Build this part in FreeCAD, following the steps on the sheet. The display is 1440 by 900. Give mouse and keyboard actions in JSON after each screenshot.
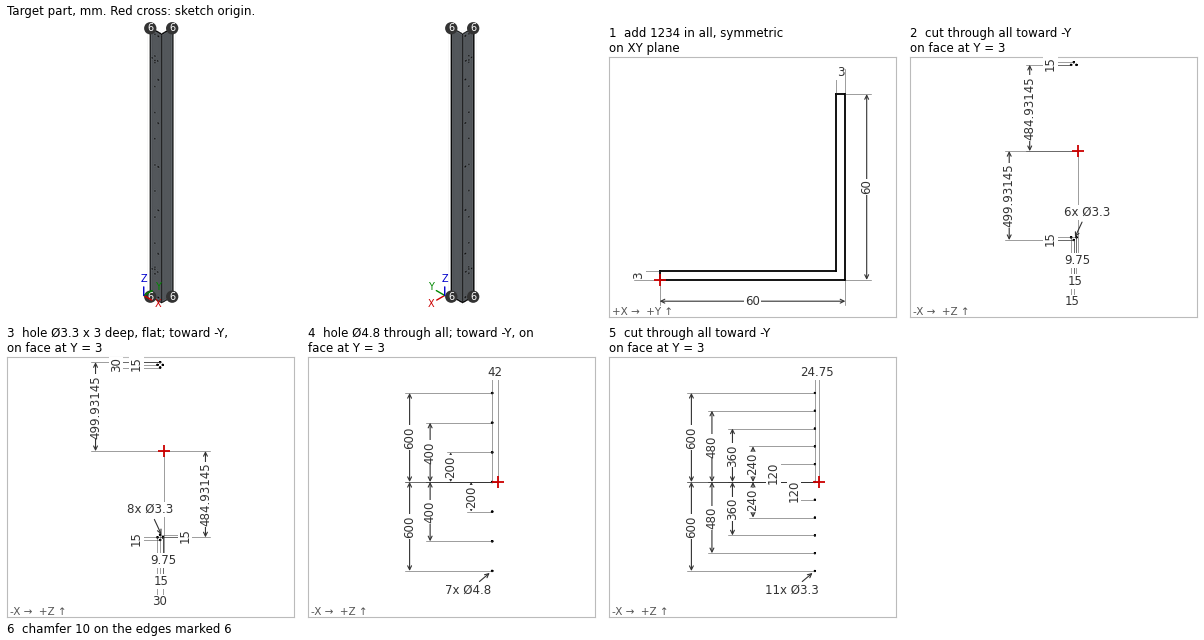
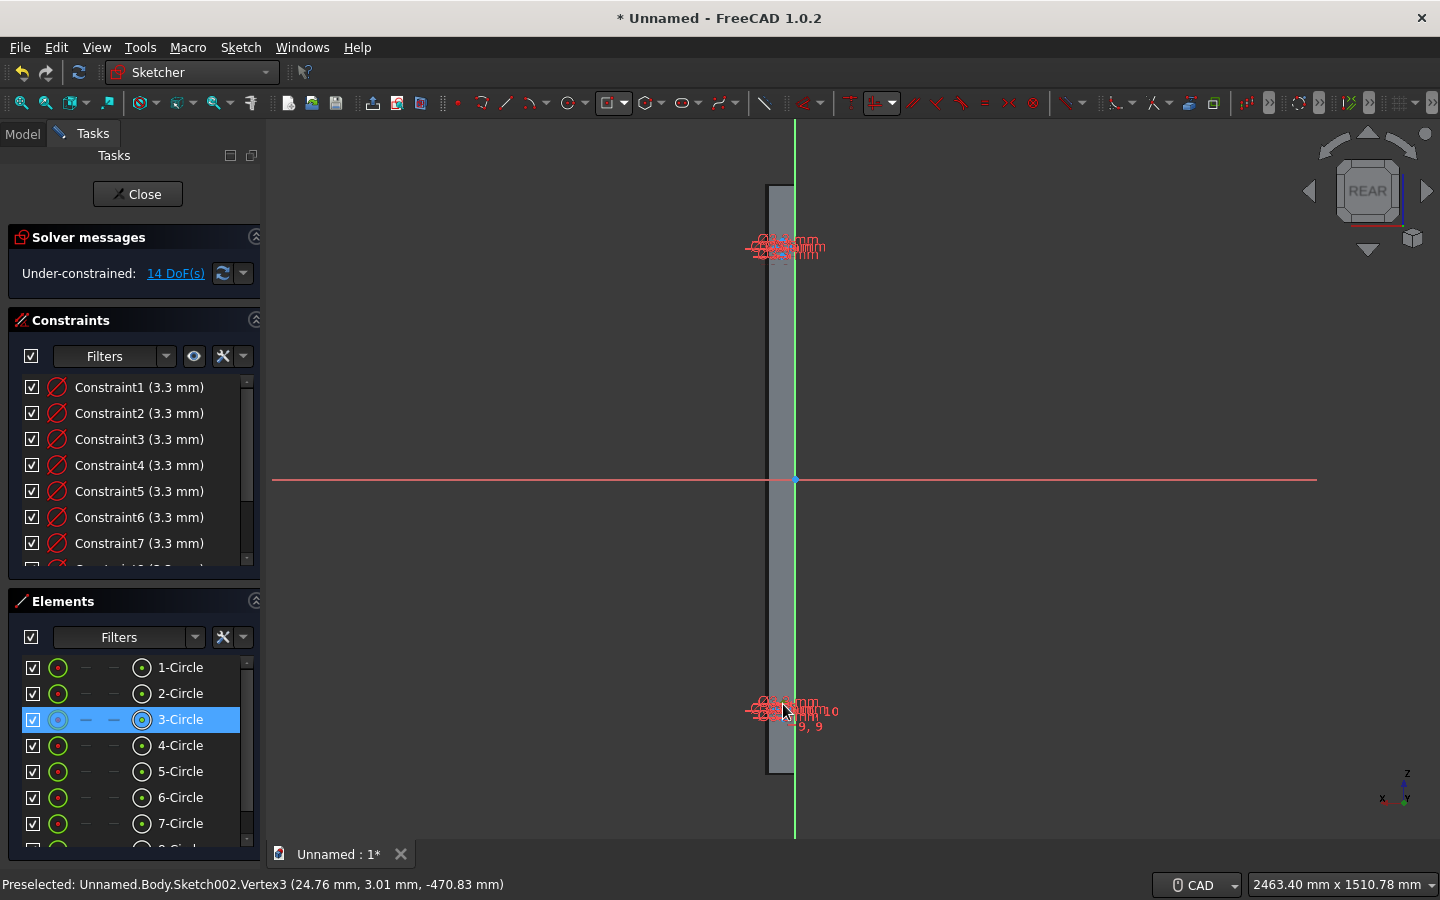
{"action": "scroll", "coordinate": [783, 242], "scroll_direction": "up", "scroll_amount": 2}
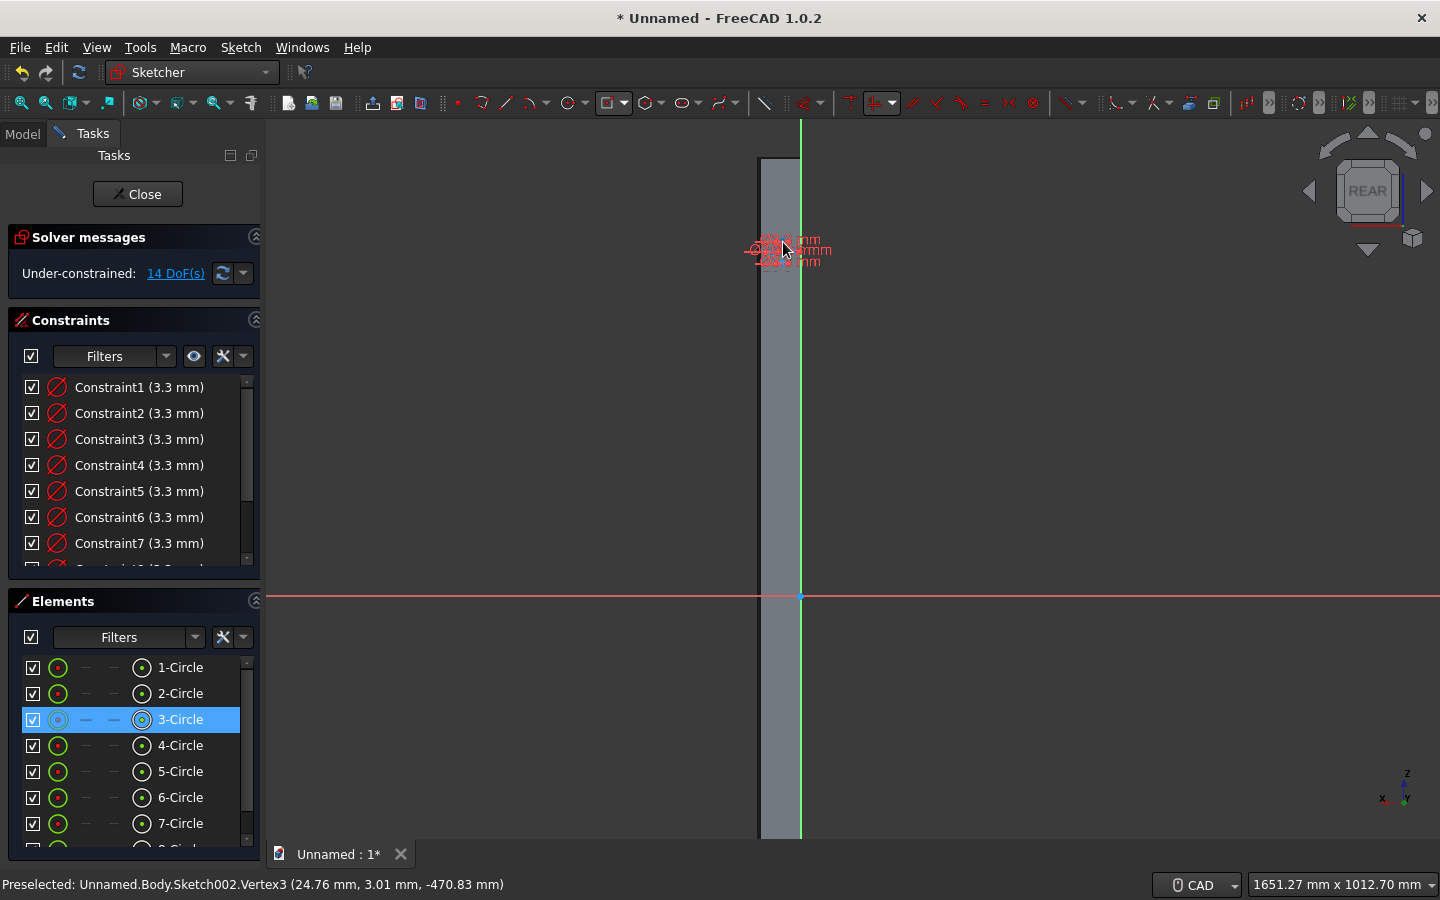
{"action": "left_click", "coordinate": [783, 242]}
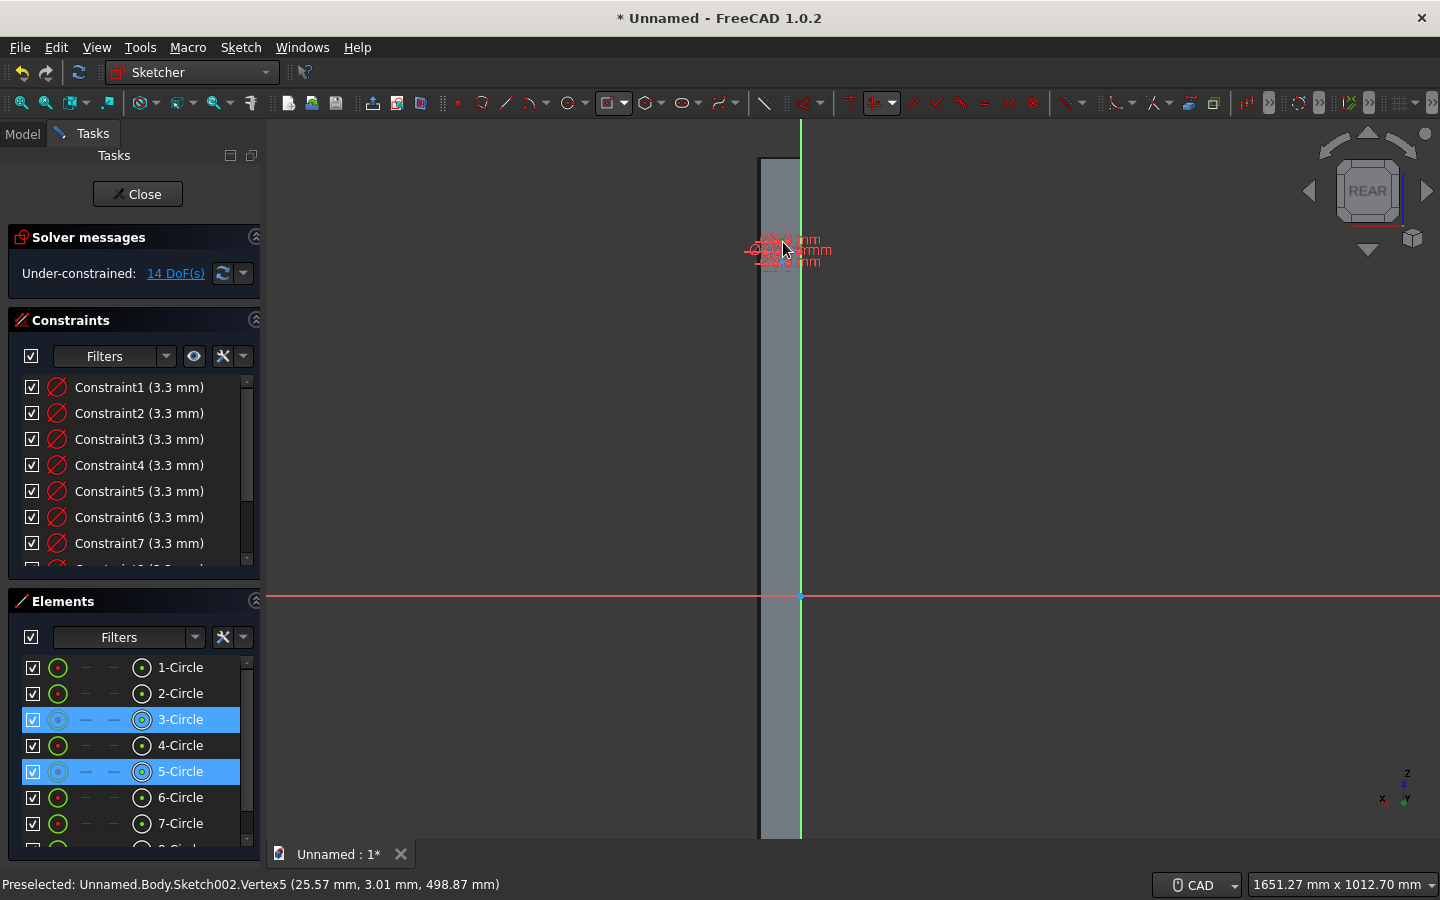
{"action": "key", "text": "v"}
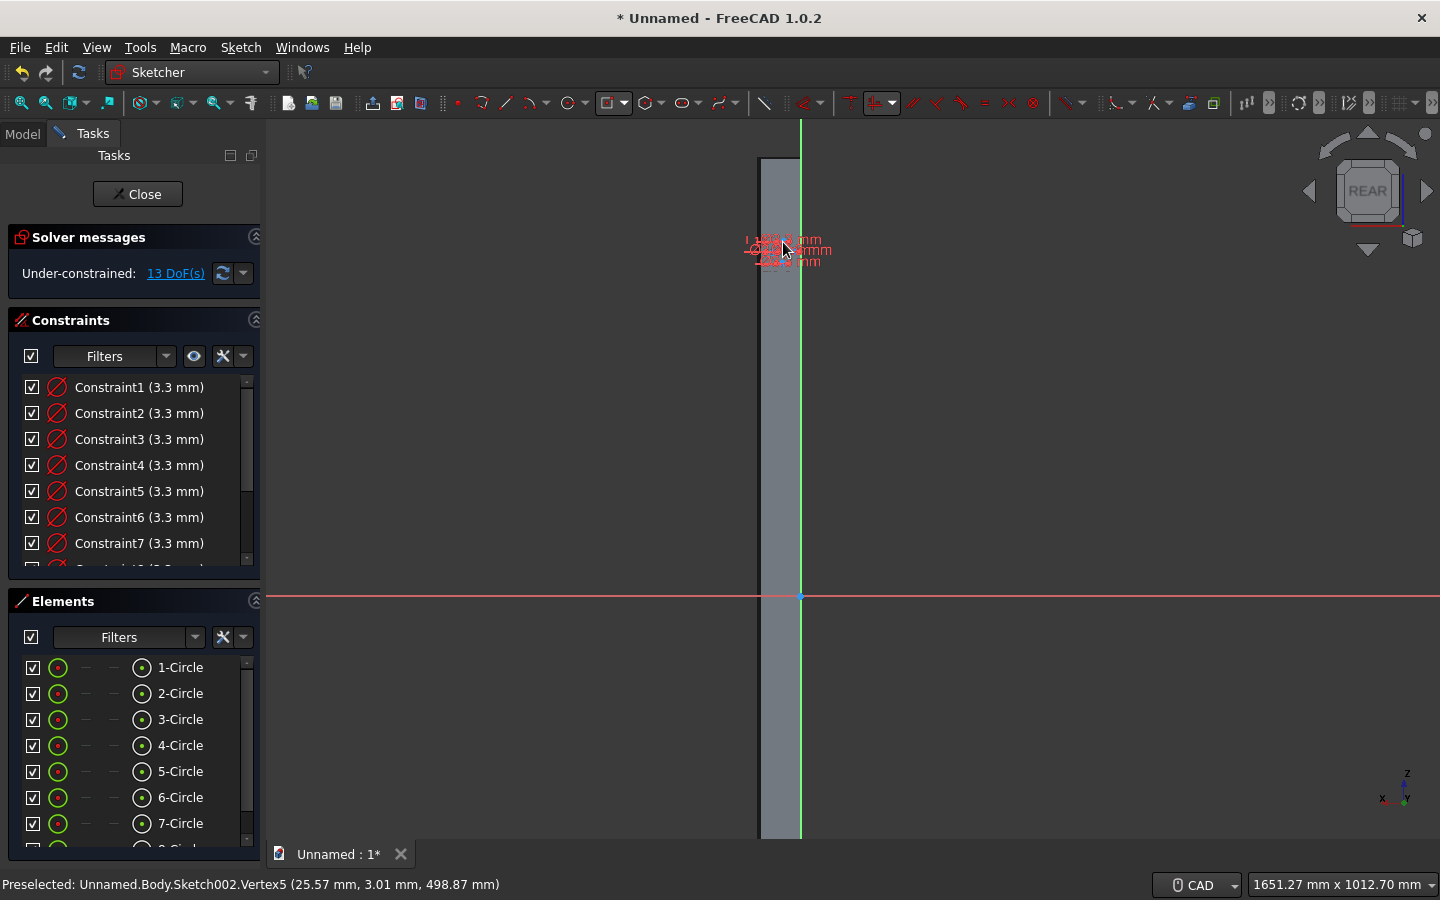
{"action": "left_click", "coordinate": [783, 242]}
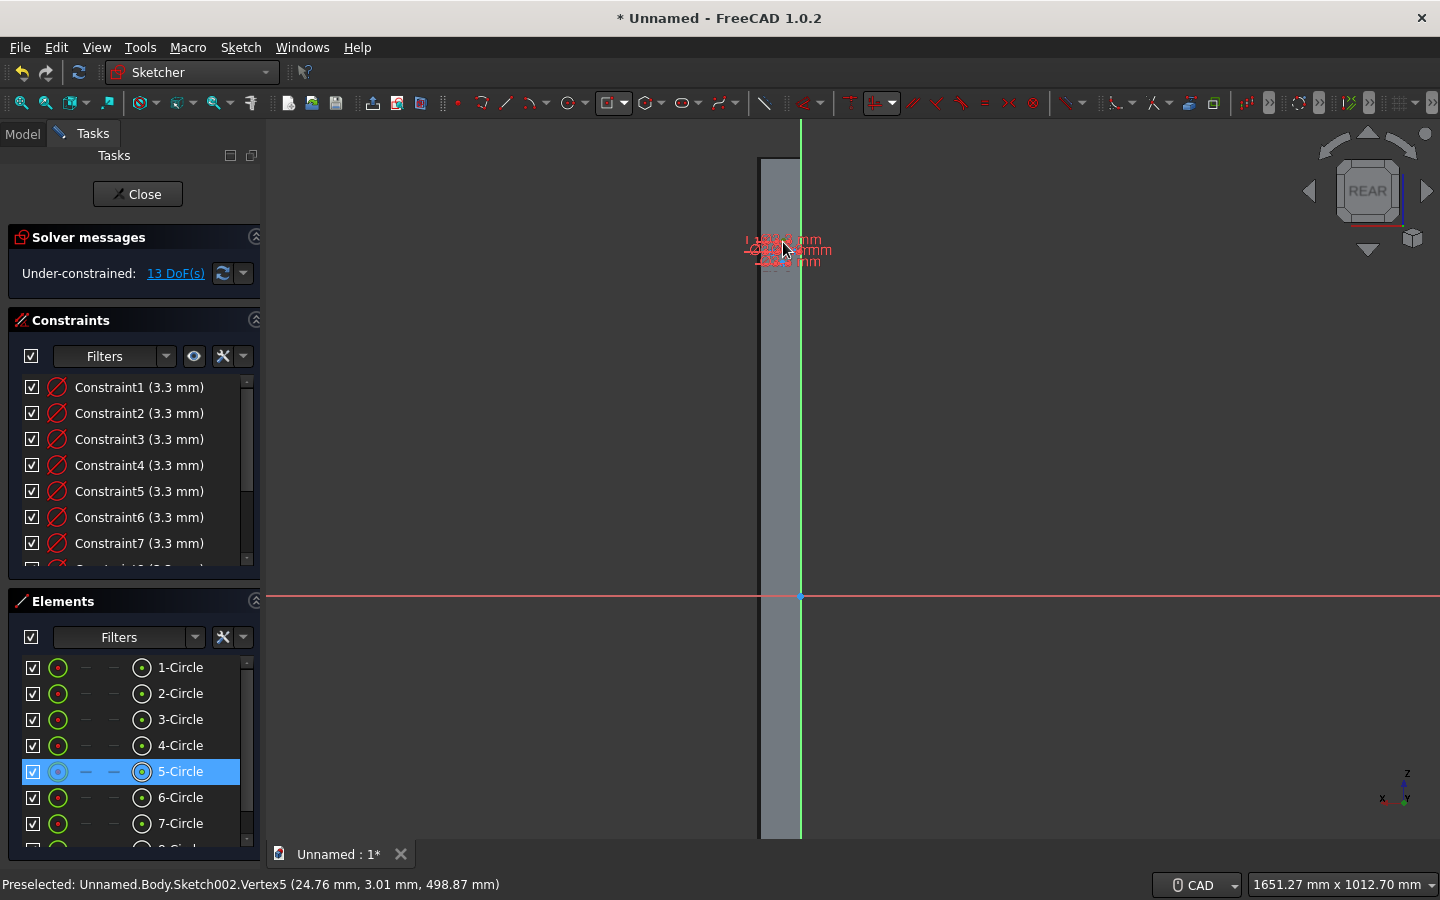
{"action": "left_click", "coordinate": [783, 264]}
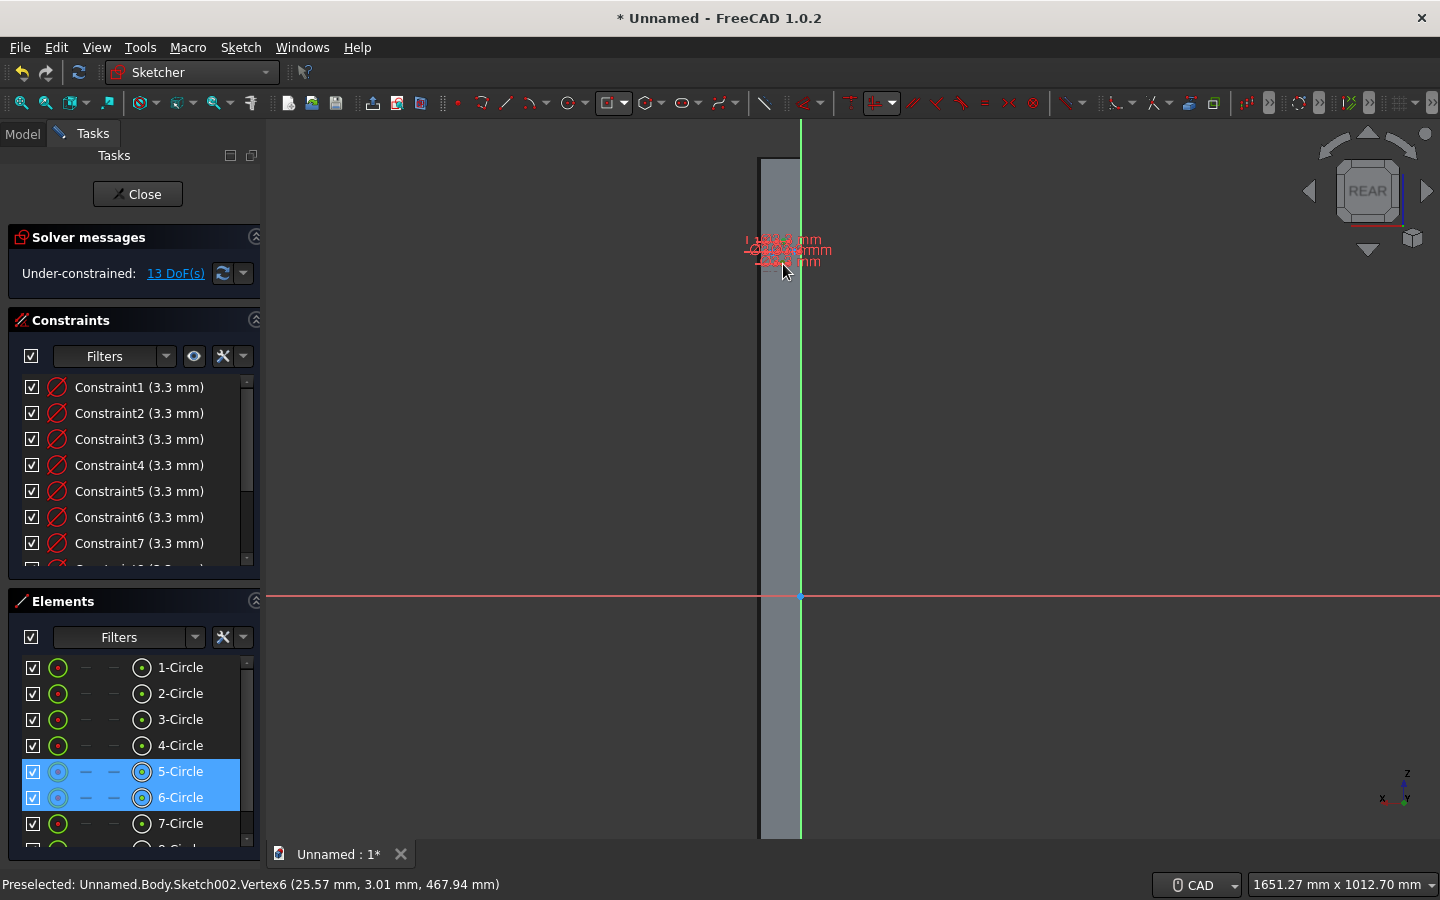
{"action": "key", "text": "v"}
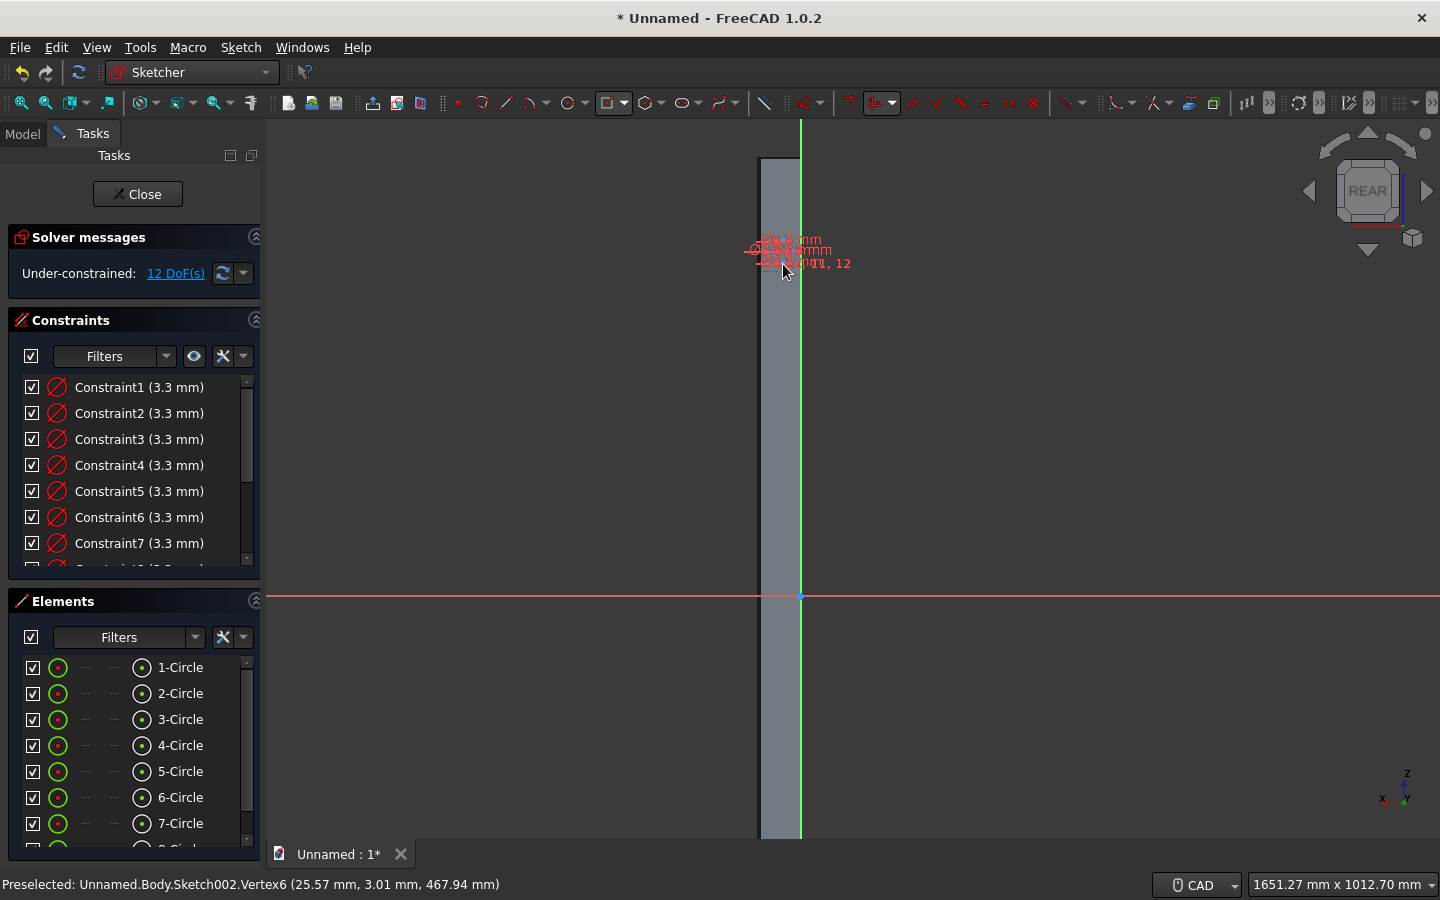
{"action": "scroll", "coordinate": [781, 241], "scroll_direction": "down", "scroll_amount": 2}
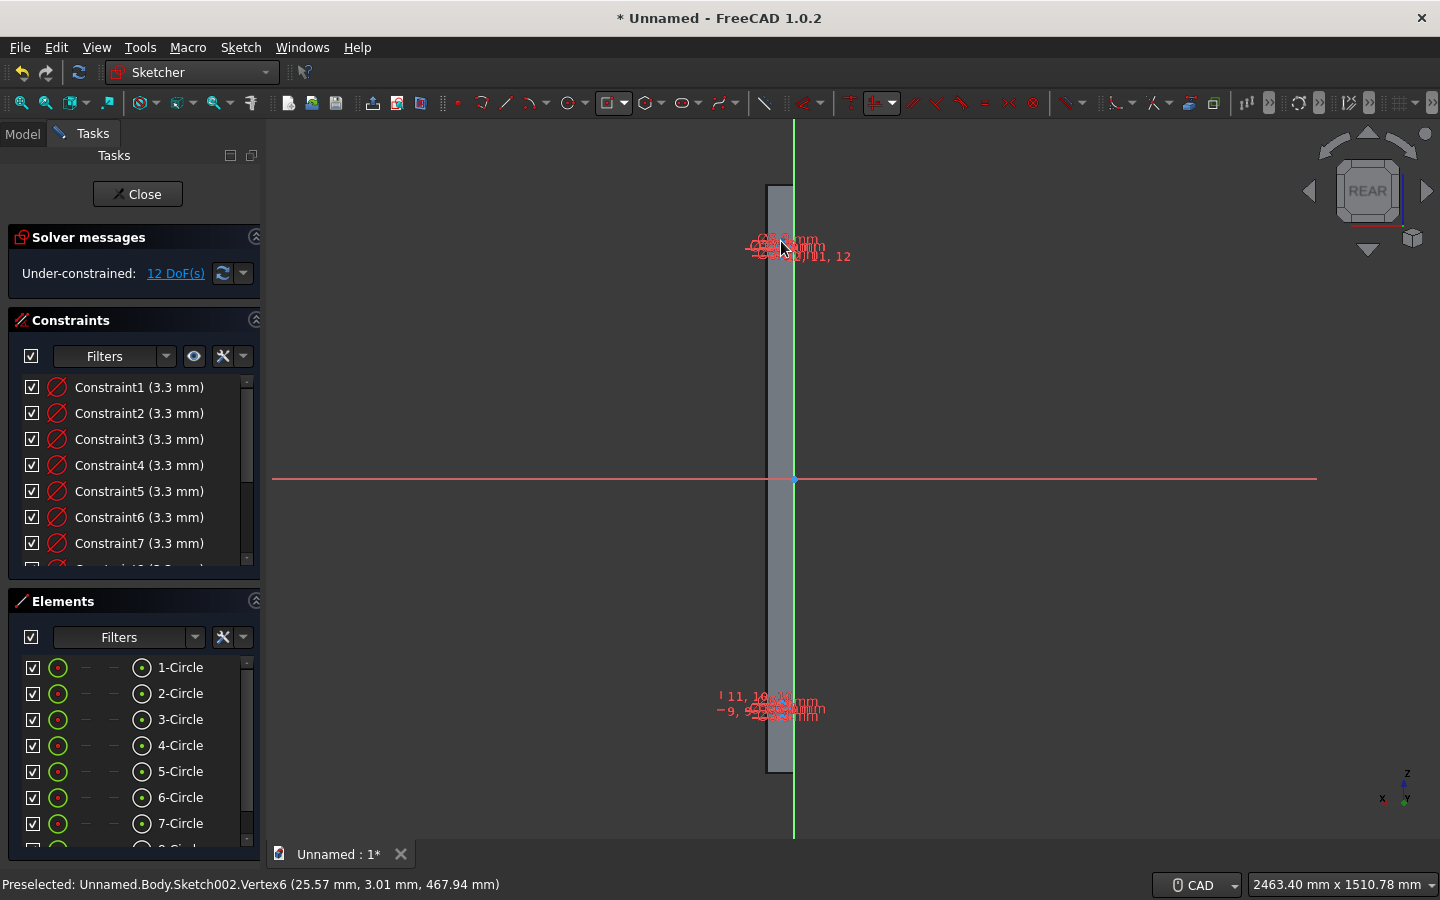
{"action": "left_click", "coordinate": [775, 711]}